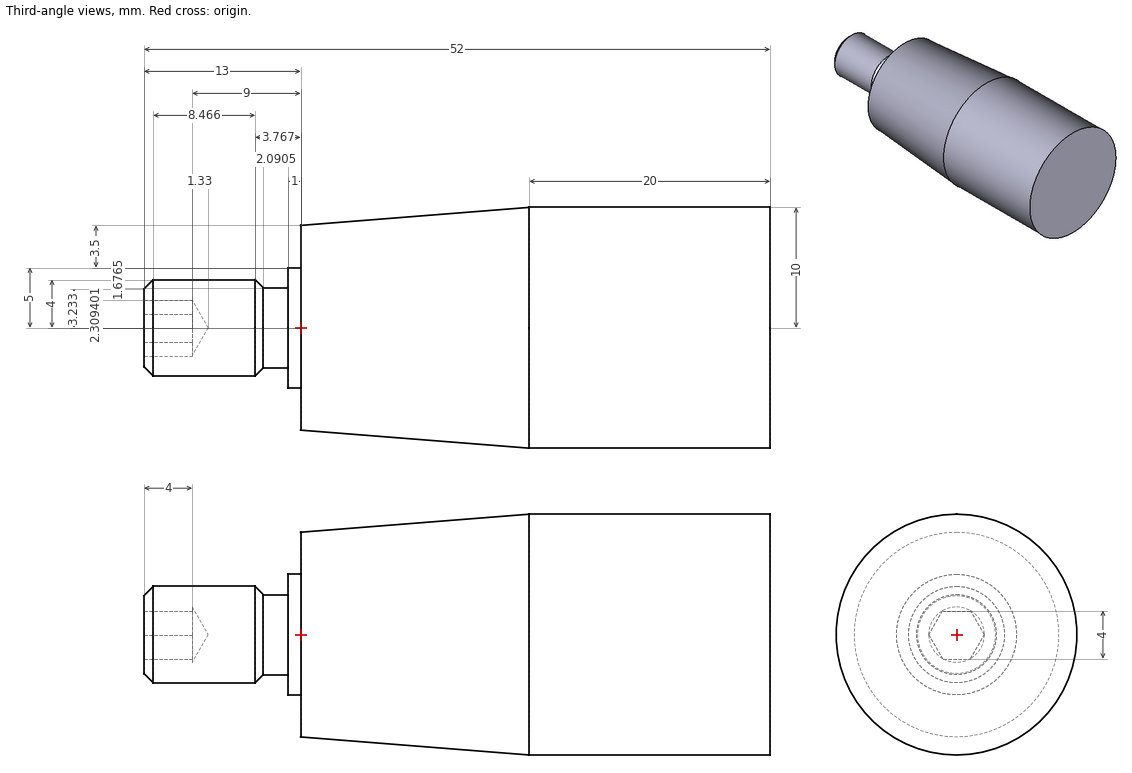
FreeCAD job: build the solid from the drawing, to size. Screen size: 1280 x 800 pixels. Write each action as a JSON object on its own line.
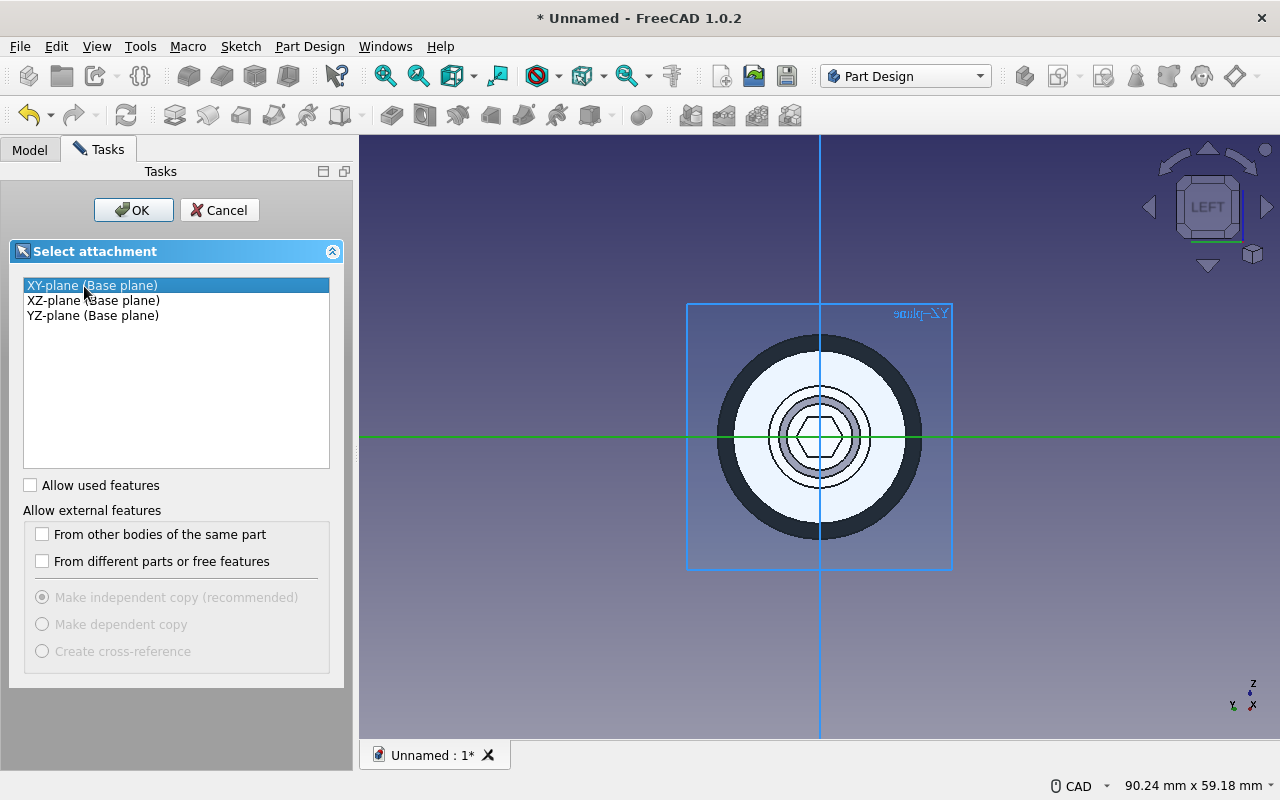
{"action": "left_click", "coordinate": [134, 210]}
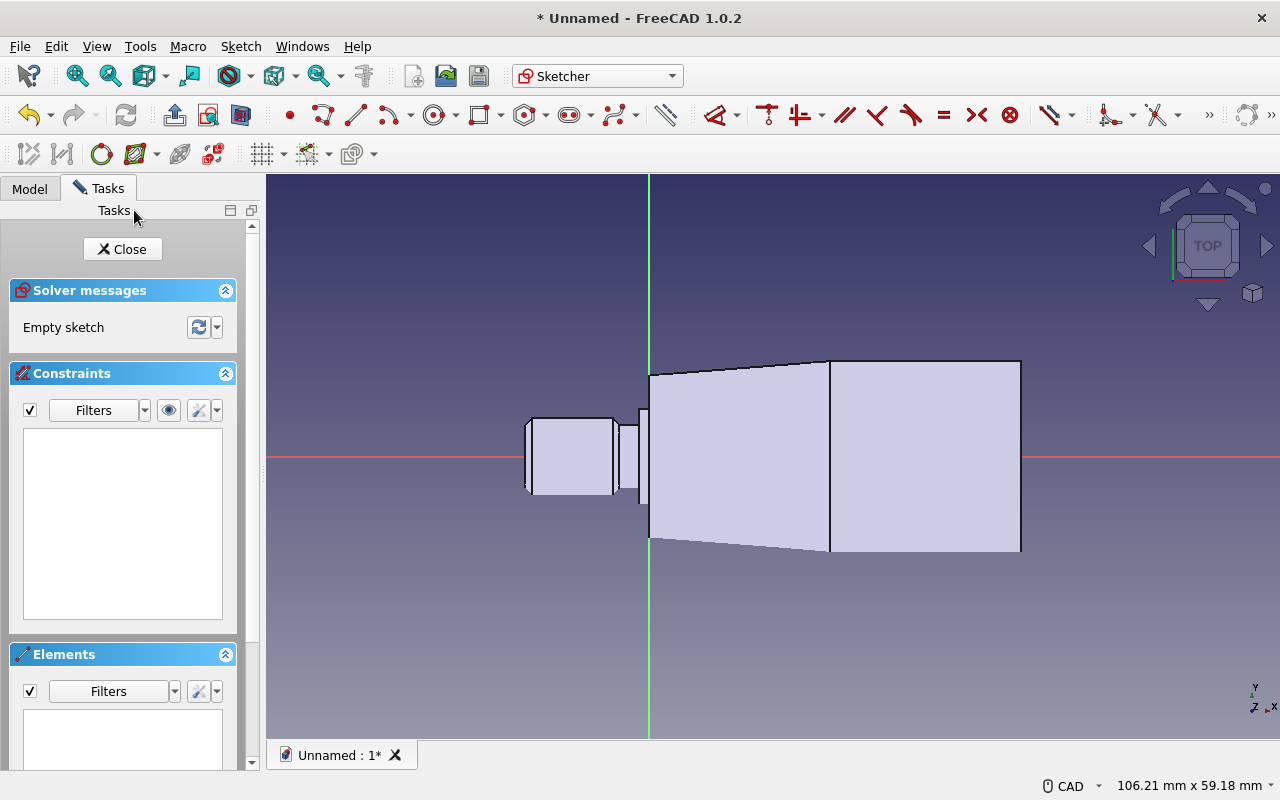
{"action": "key", "text": "q s"}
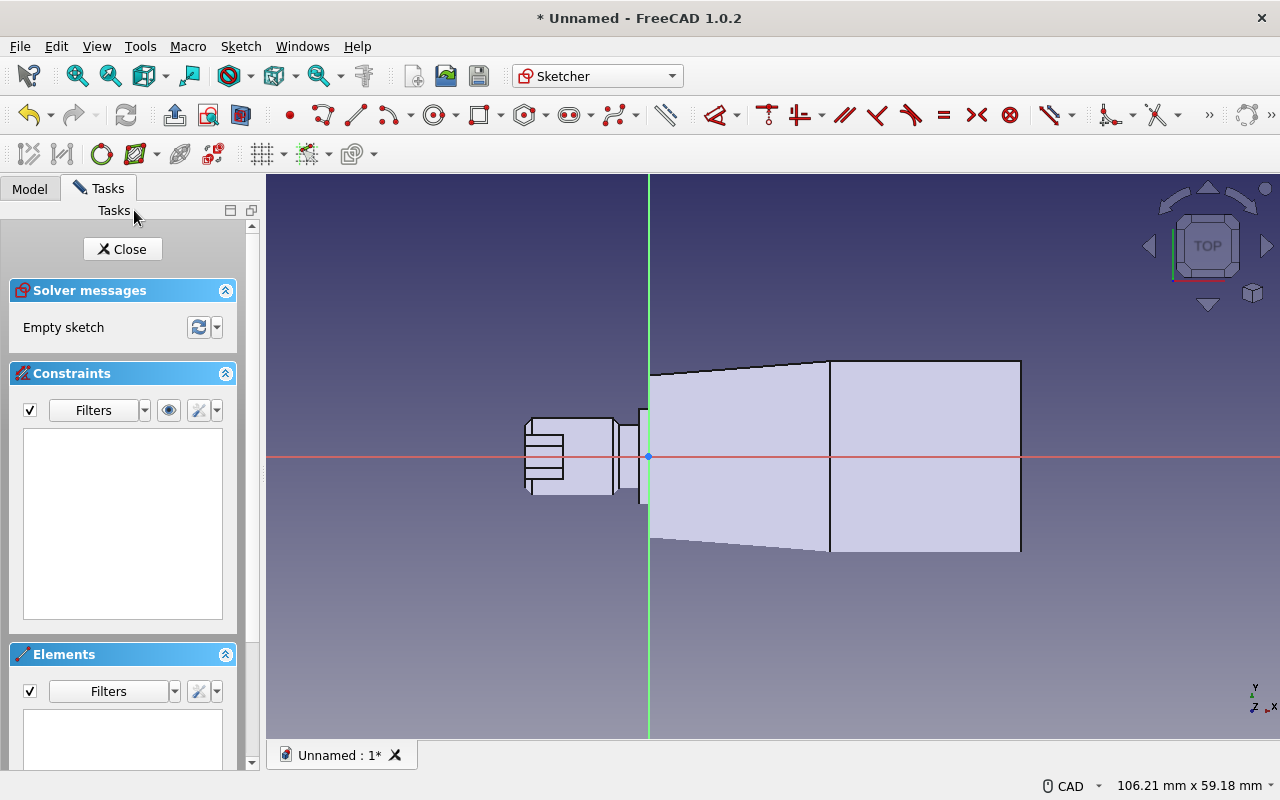
{"action": "scroll", "coordinate": [561, 445], "scroll_direction": "up", "scroll_amount": 14}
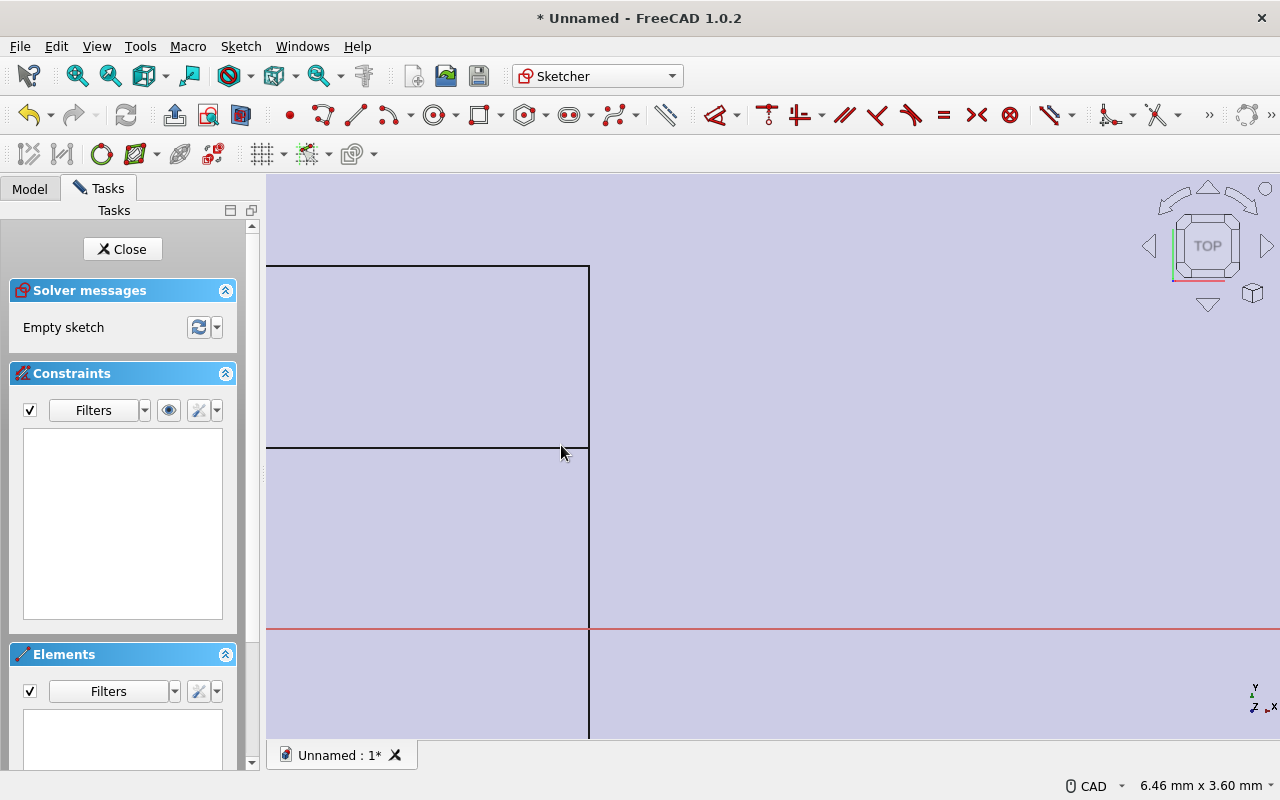
{"action": "left_click", "coordinate": [323, 116]}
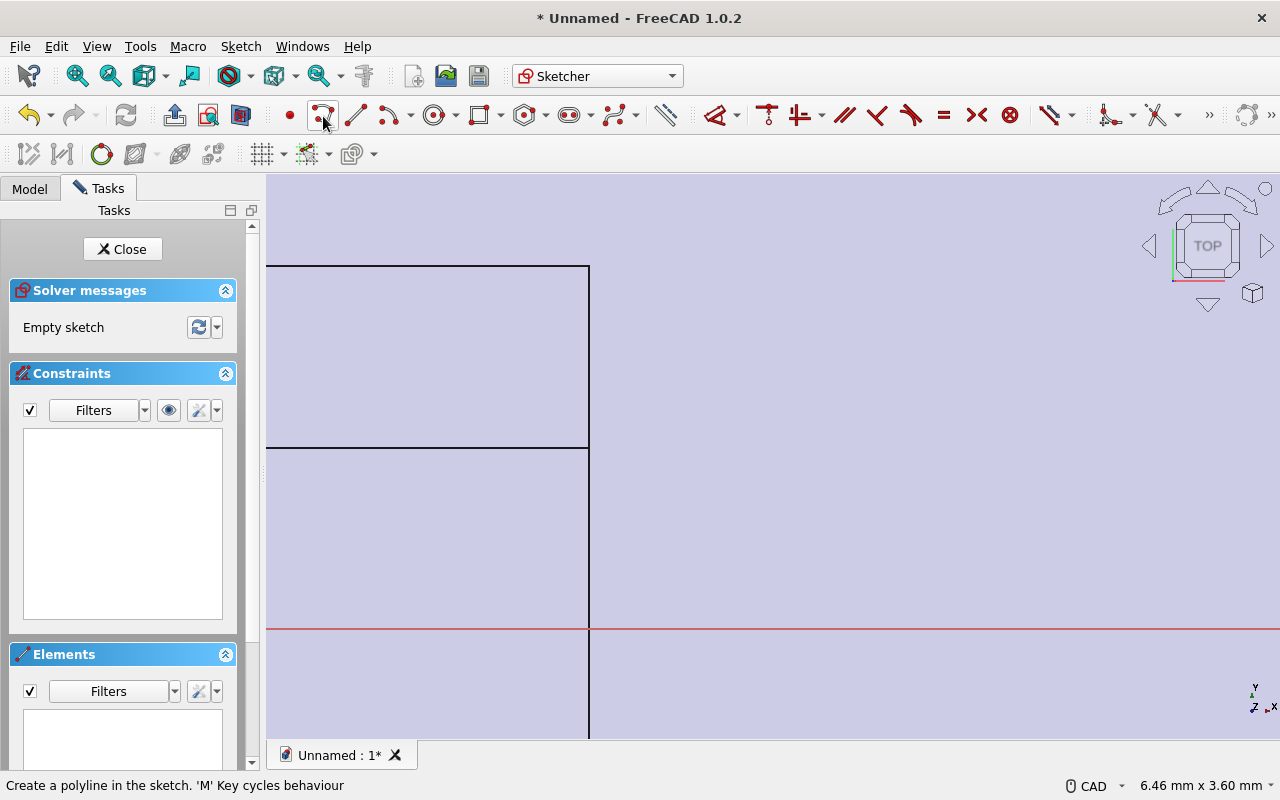
{"action": "left_click", "coordinate": [798, 629]}
{"action": "left_click", "coordinate": [589, 266]}
{"action": "left_click", "coordinate": [589, 620]}
{"action": "left_click", "coordinate": [798, 629]}
{"action": "key", "text": "Escape"}
{"action": "key", "text": "Escape"}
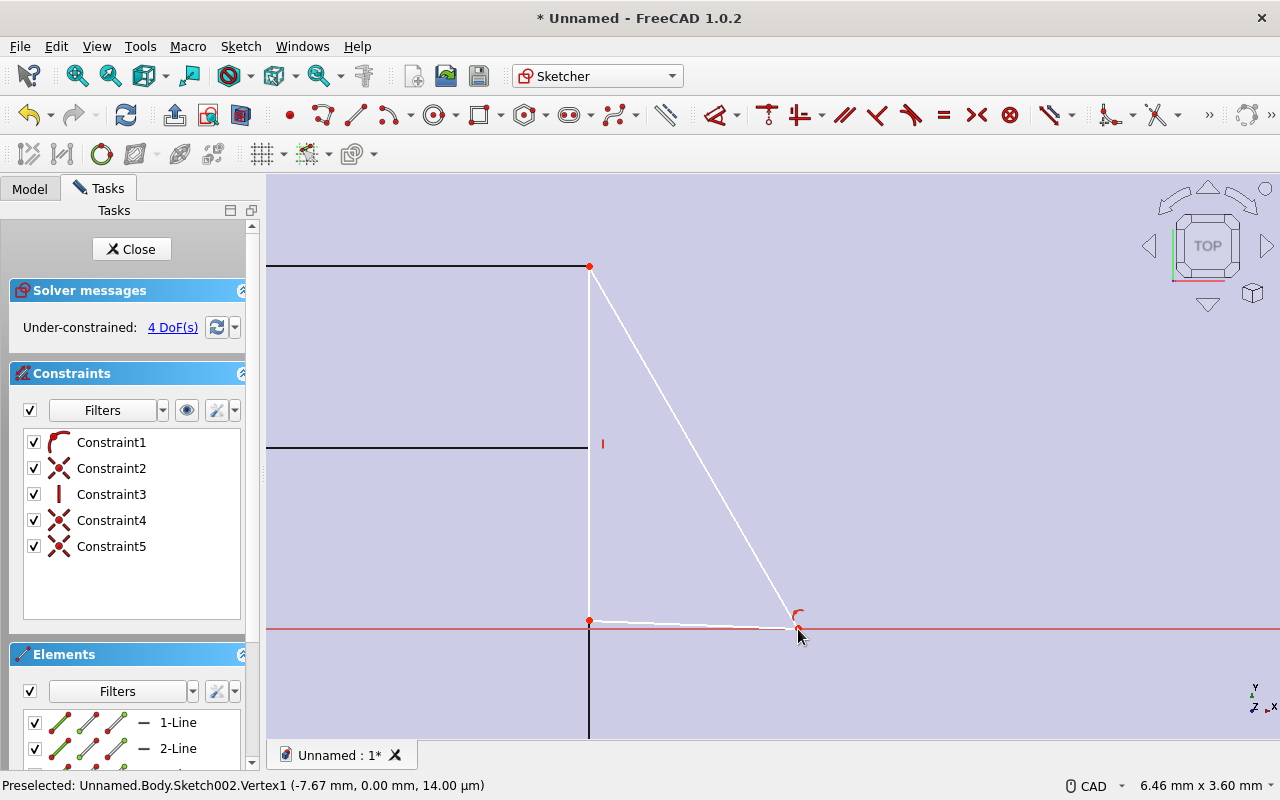
{"action": "left_click", "coordinate": [735, 627]}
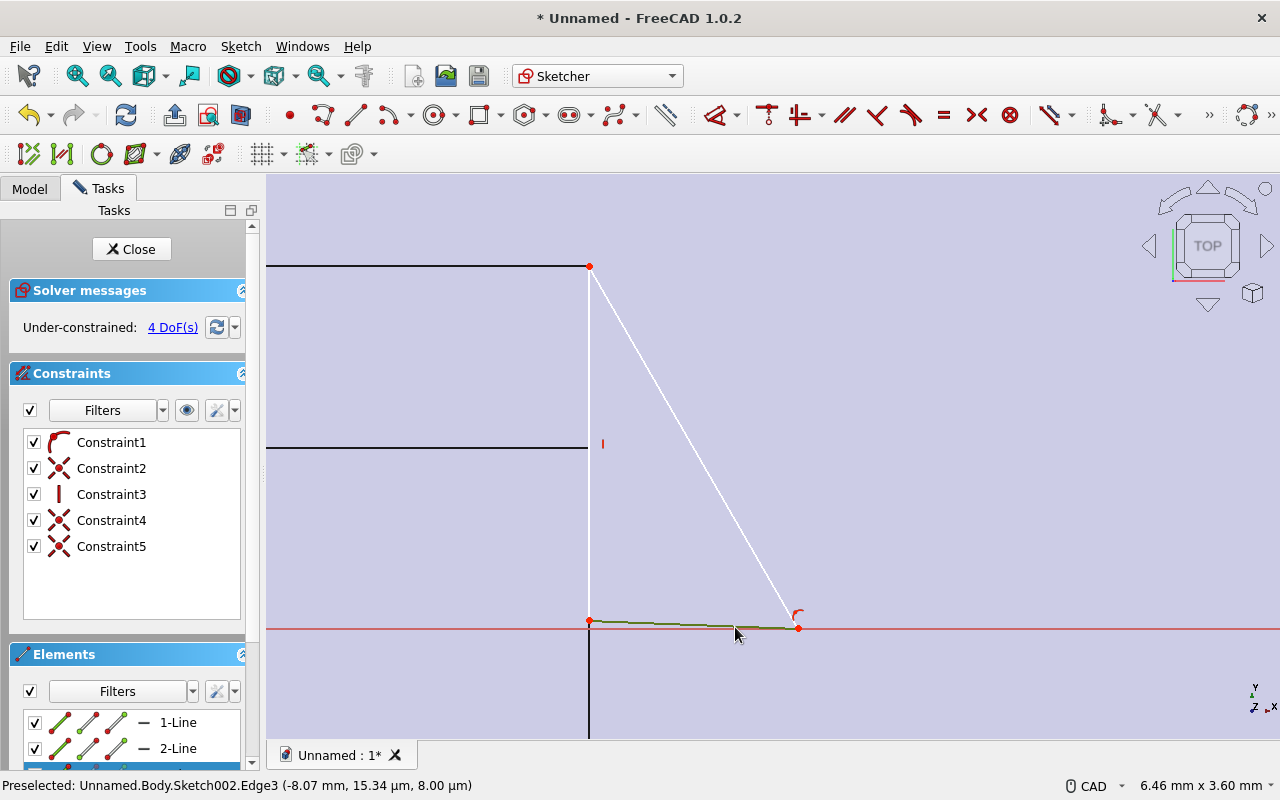
{"action": "key", "text": "h"}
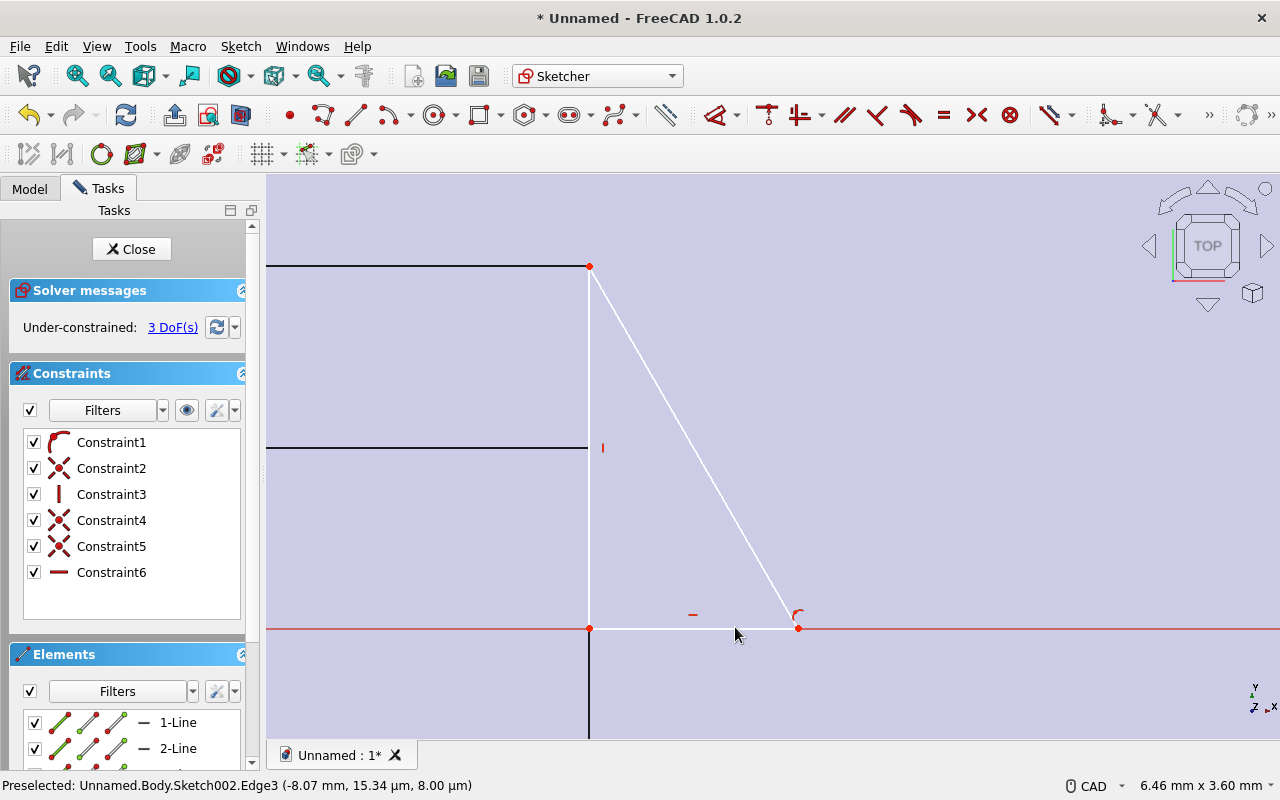
{"action": "key", "text": "d"}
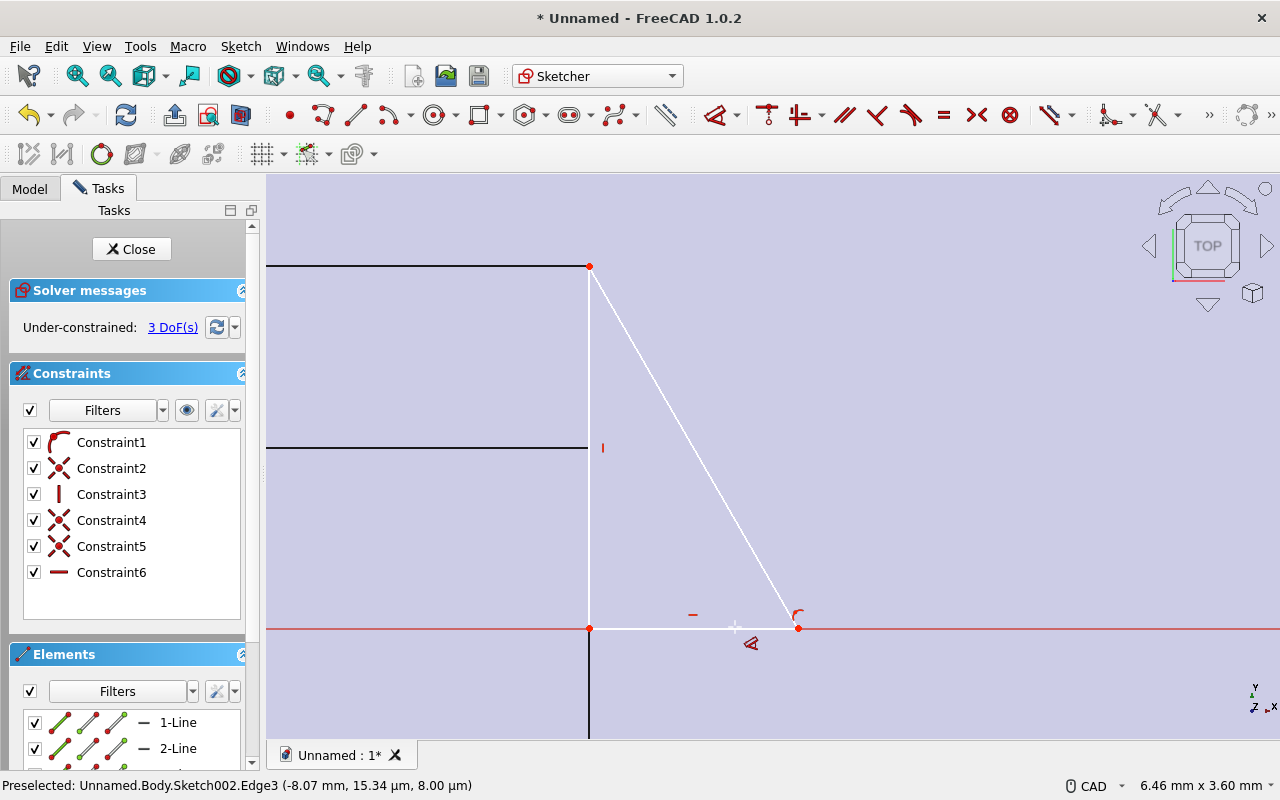
{"action": "left_click", "coordinate": [589, 267]}
{"action": "left_click", "coordinate": [852, 663]}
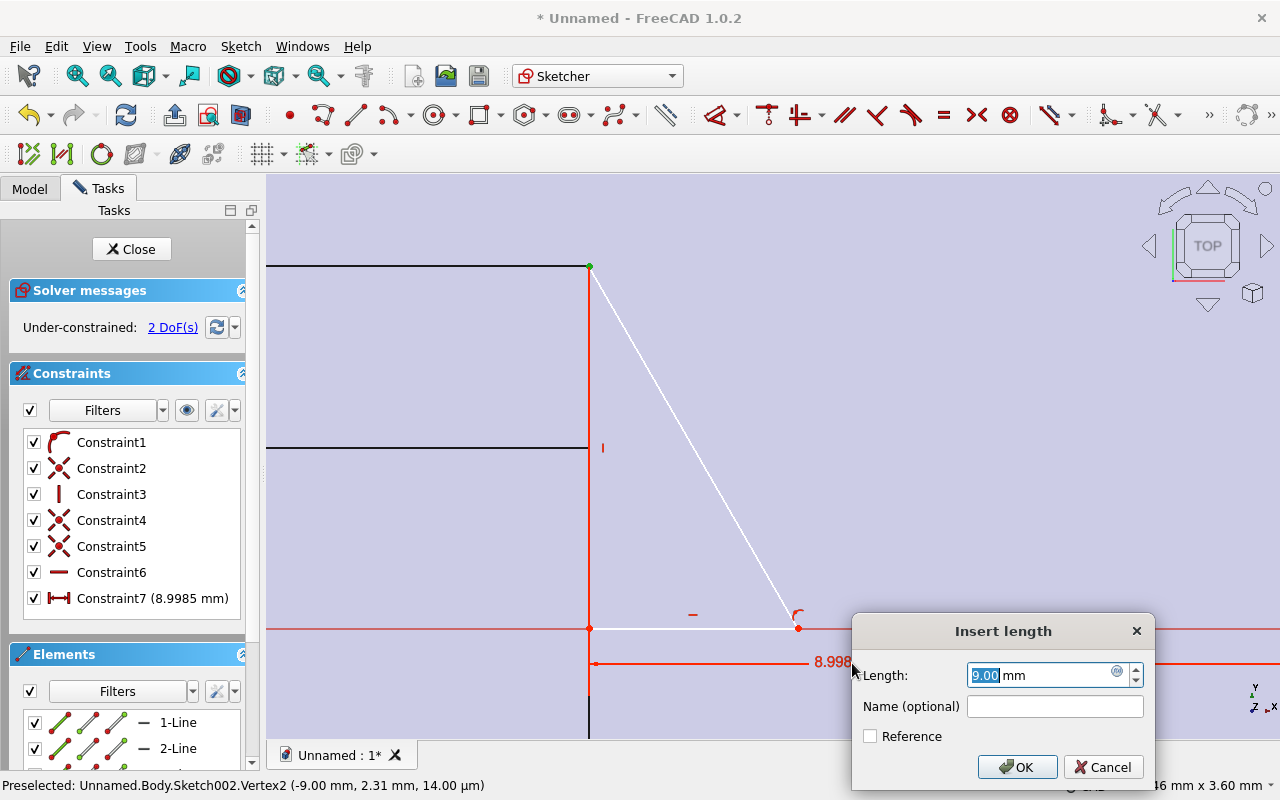
{"action": "type", "text": "9"}
{"action": "key", "text": "Return"}